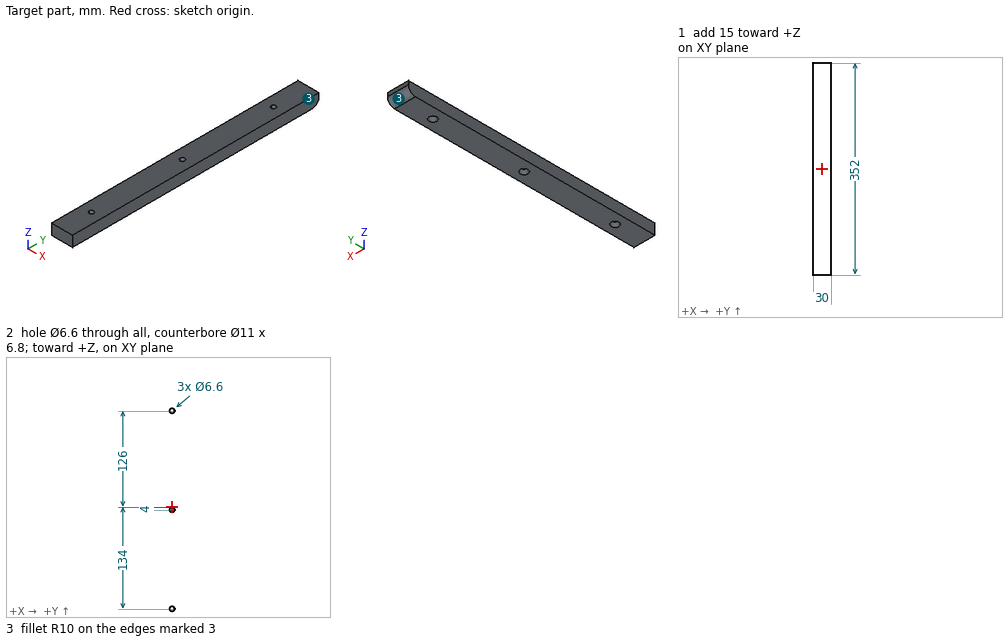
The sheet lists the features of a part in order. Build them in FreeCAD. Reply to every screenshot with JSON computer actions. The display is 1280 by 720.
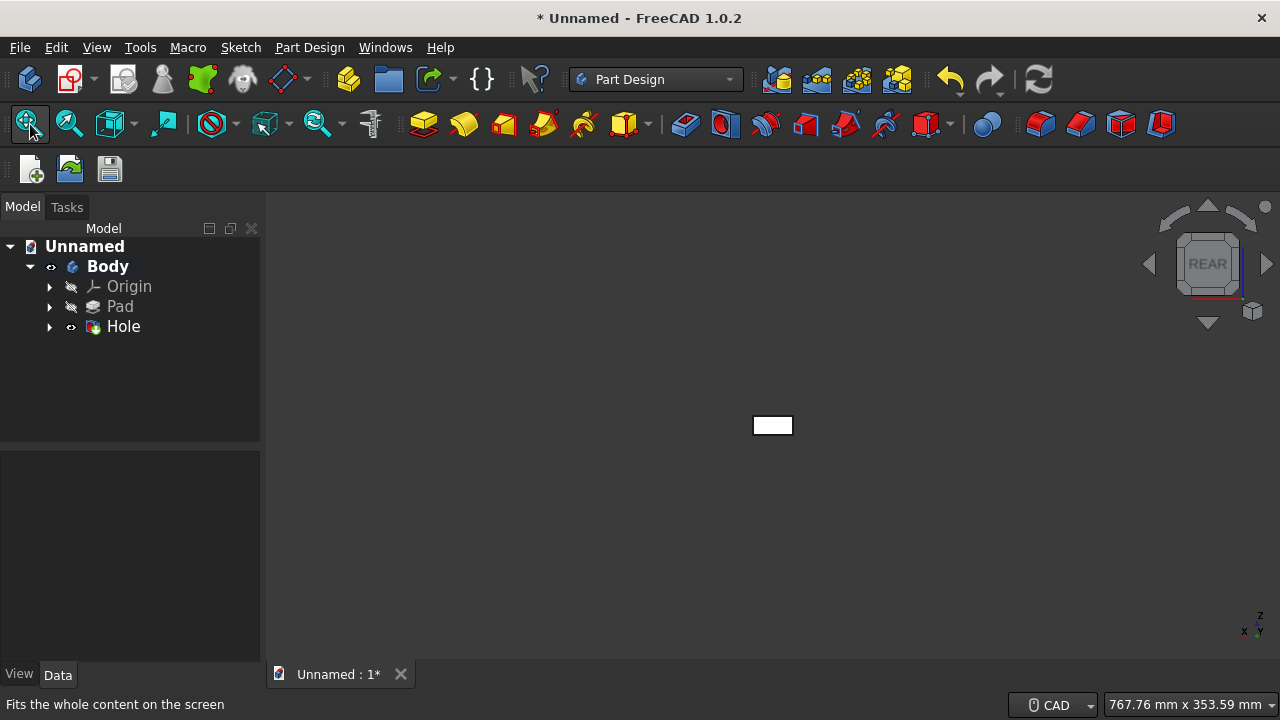
{"action": "left_click", "coordinate": [773, 434]}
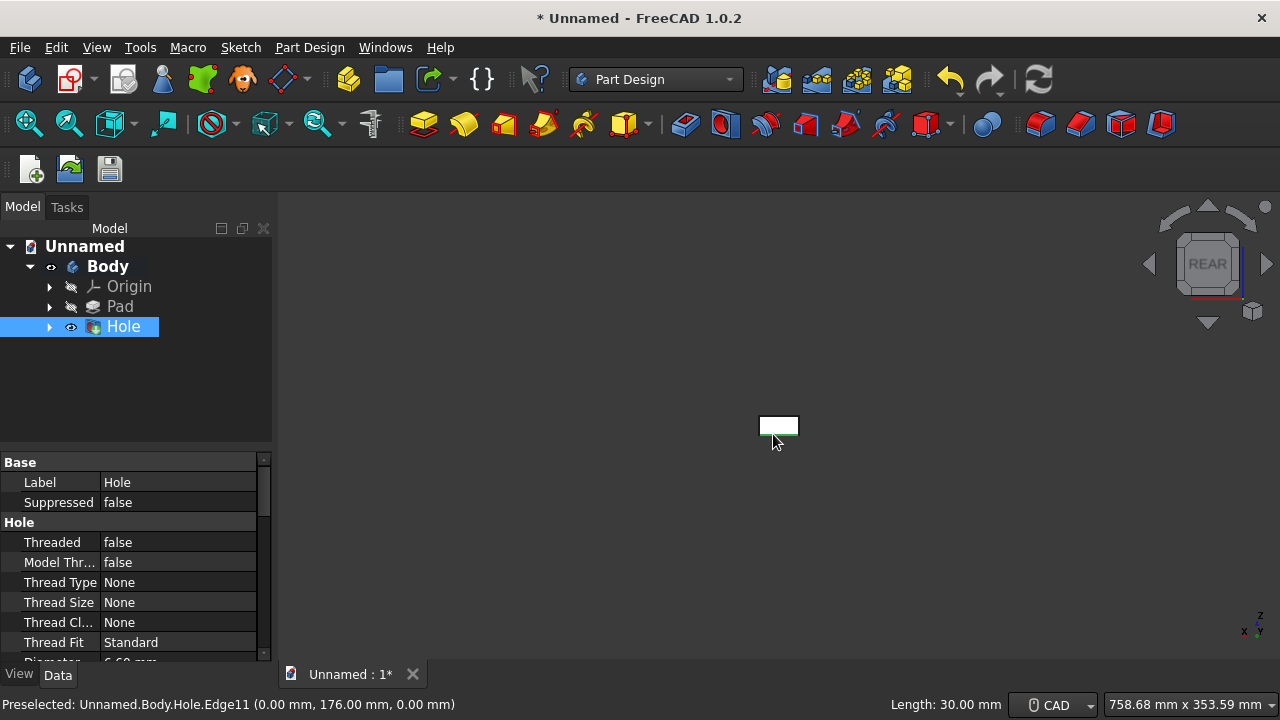
{"action": "left_click", "coordinate": [1042, 124]}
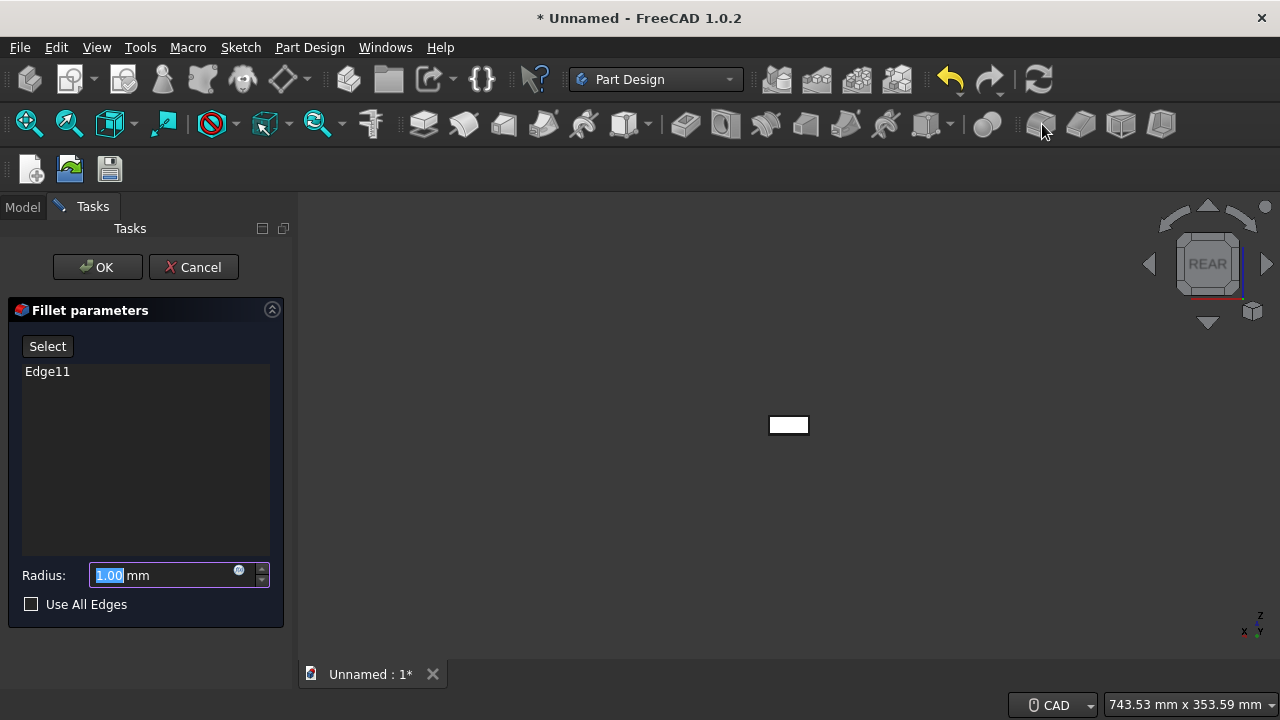
{"action": "type", "text": "10"}
{"action": "key", "text": "Tab"}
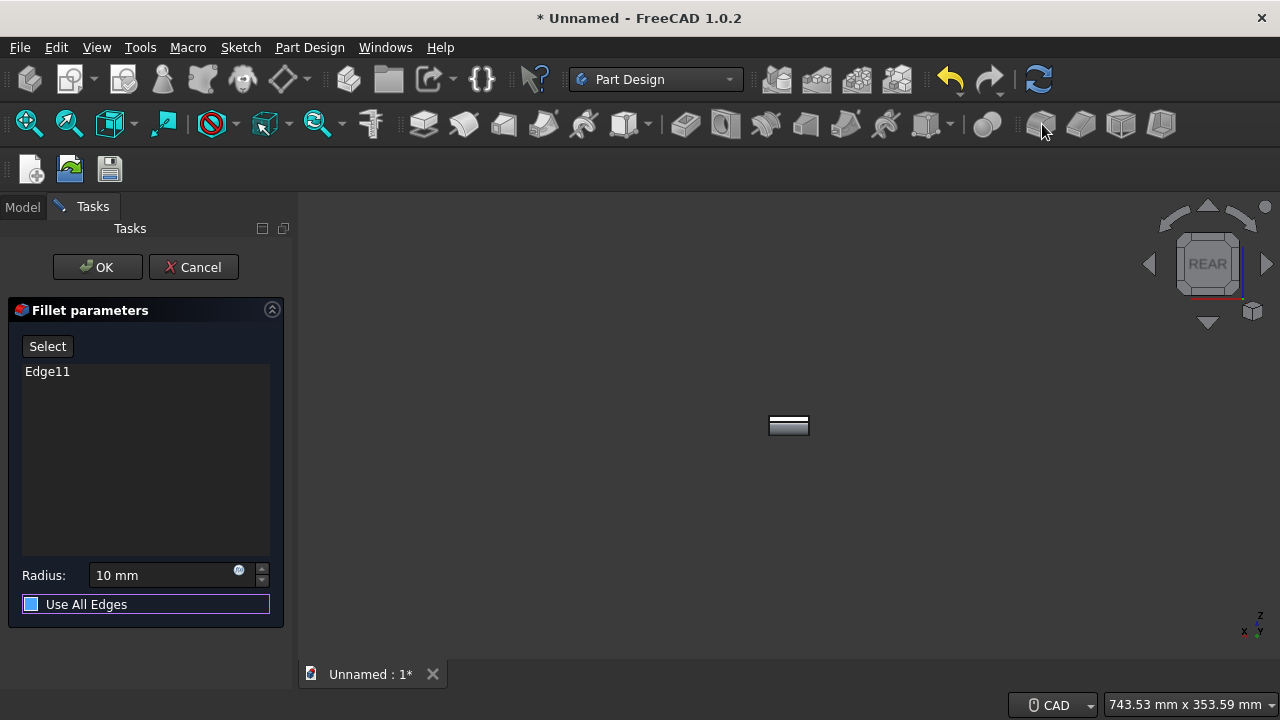
{"action": "left_click", "coordinate": [98, 267]}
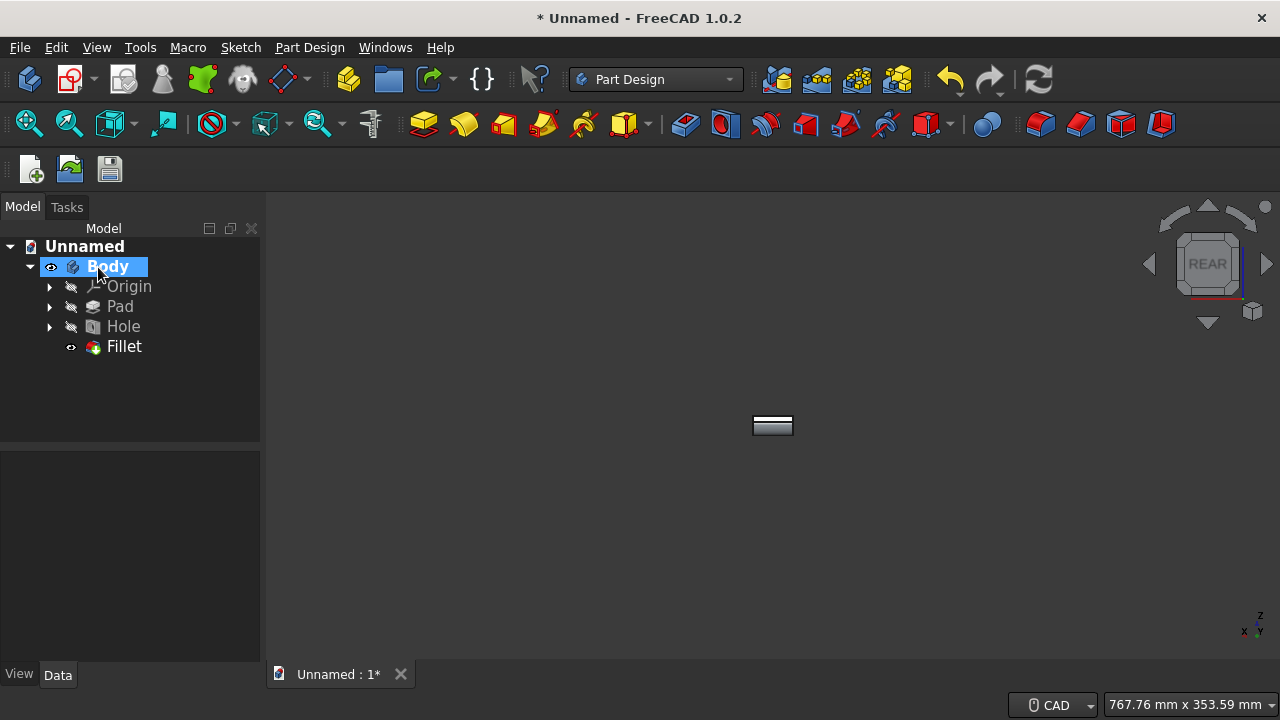
{"action": "key", "text": "0"}